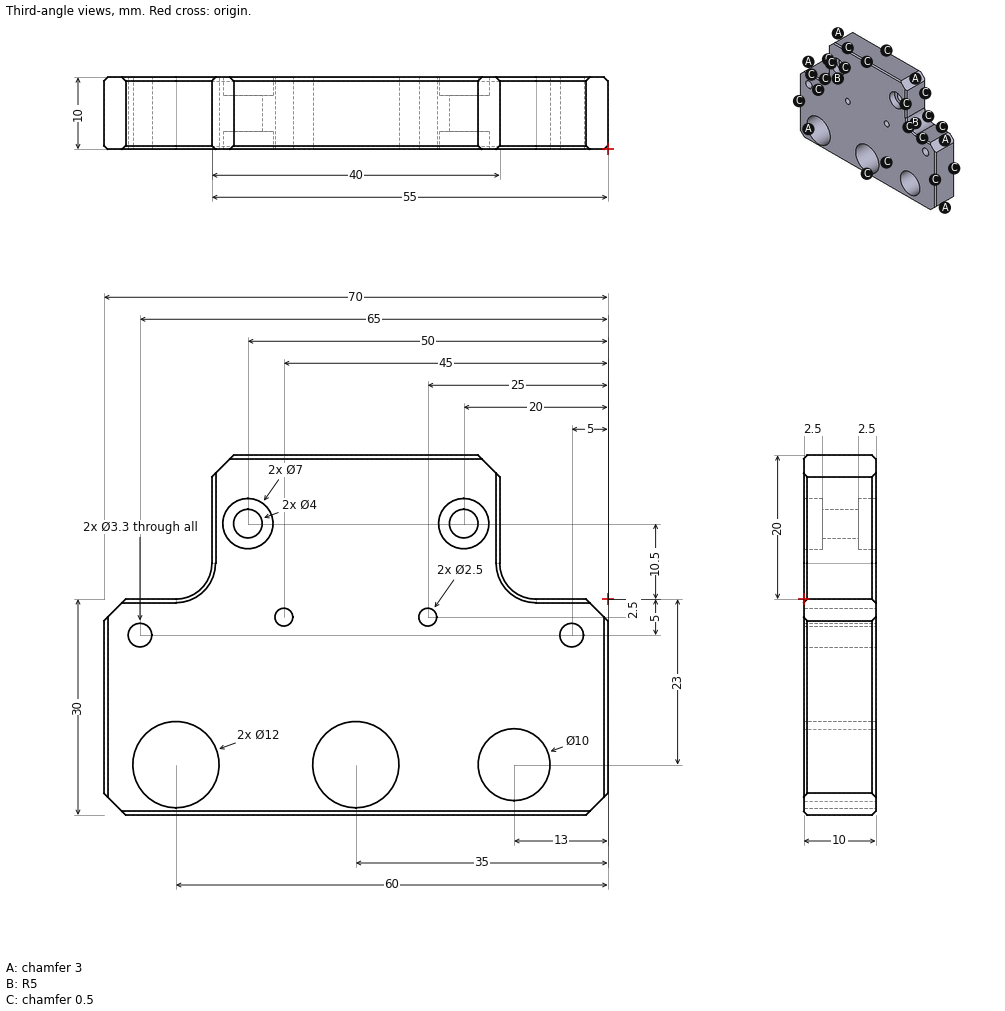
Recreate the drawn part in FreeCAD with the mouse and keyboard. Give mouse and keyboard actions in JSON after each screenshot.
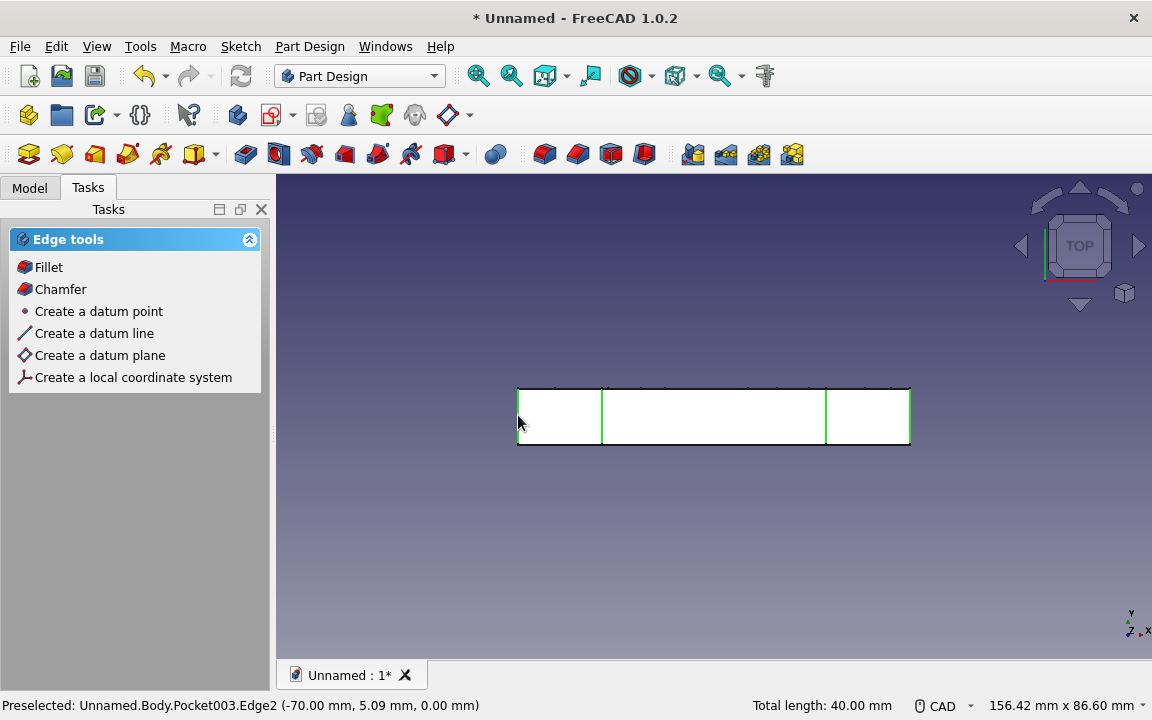
{"action": "key", "text": "1"}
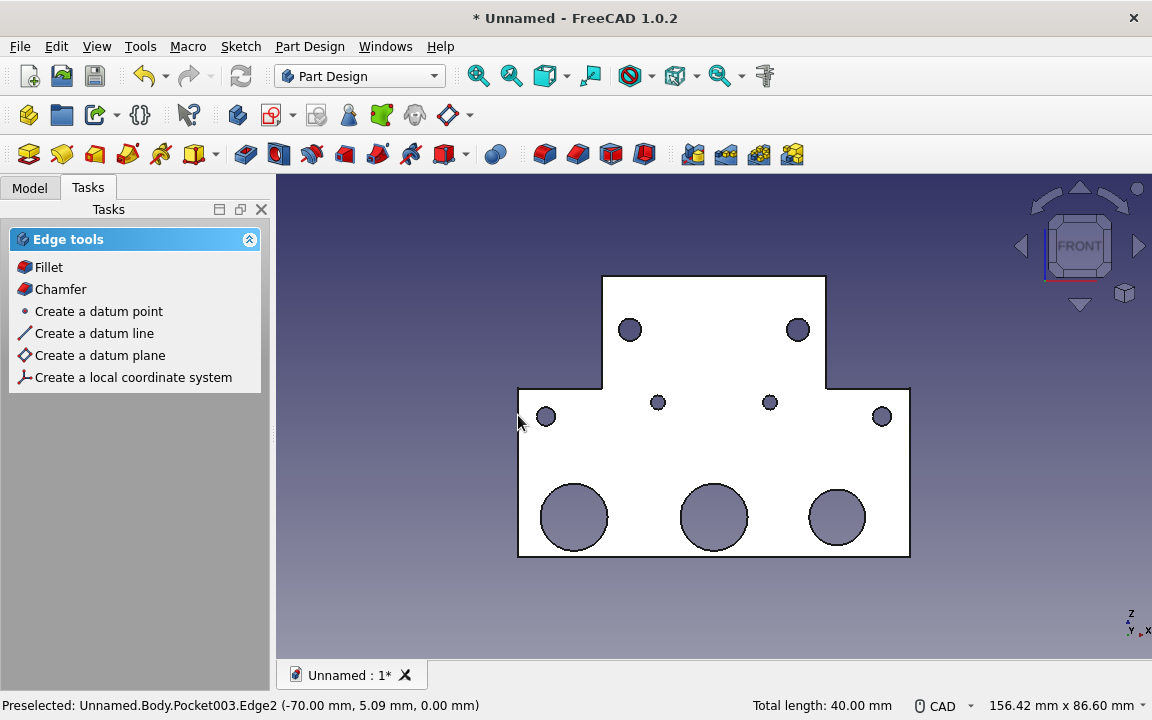
{"action": "key", "text": "3"}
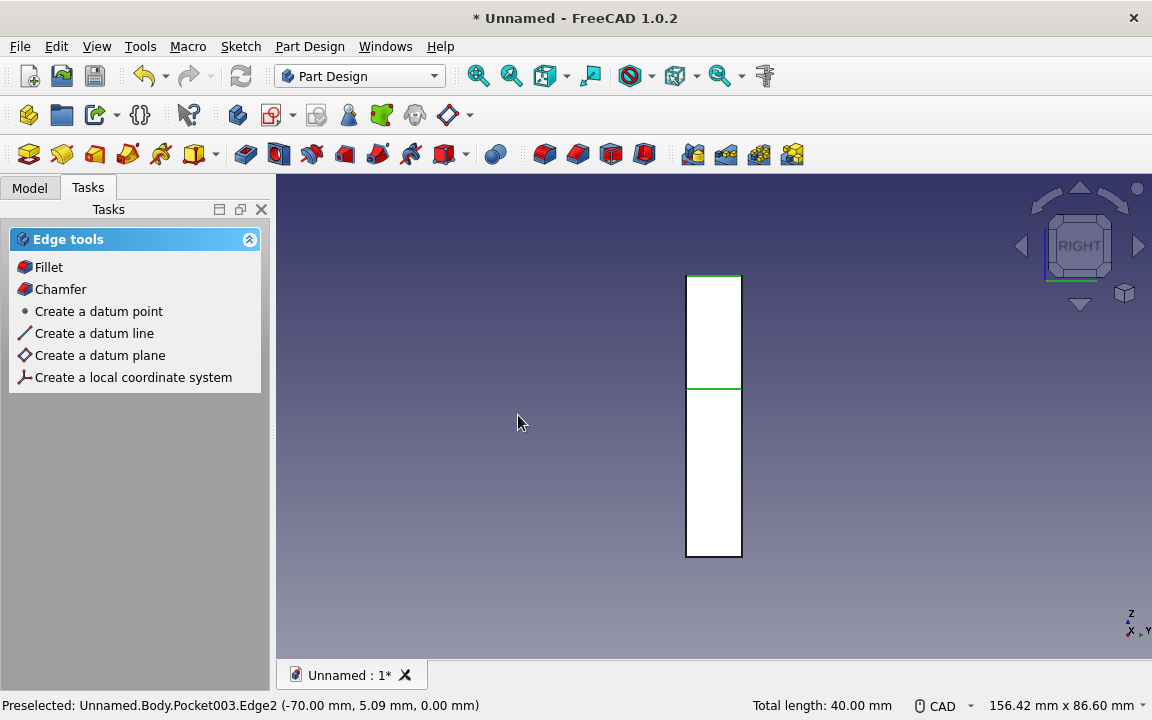
{"action": "key", "text": "5"}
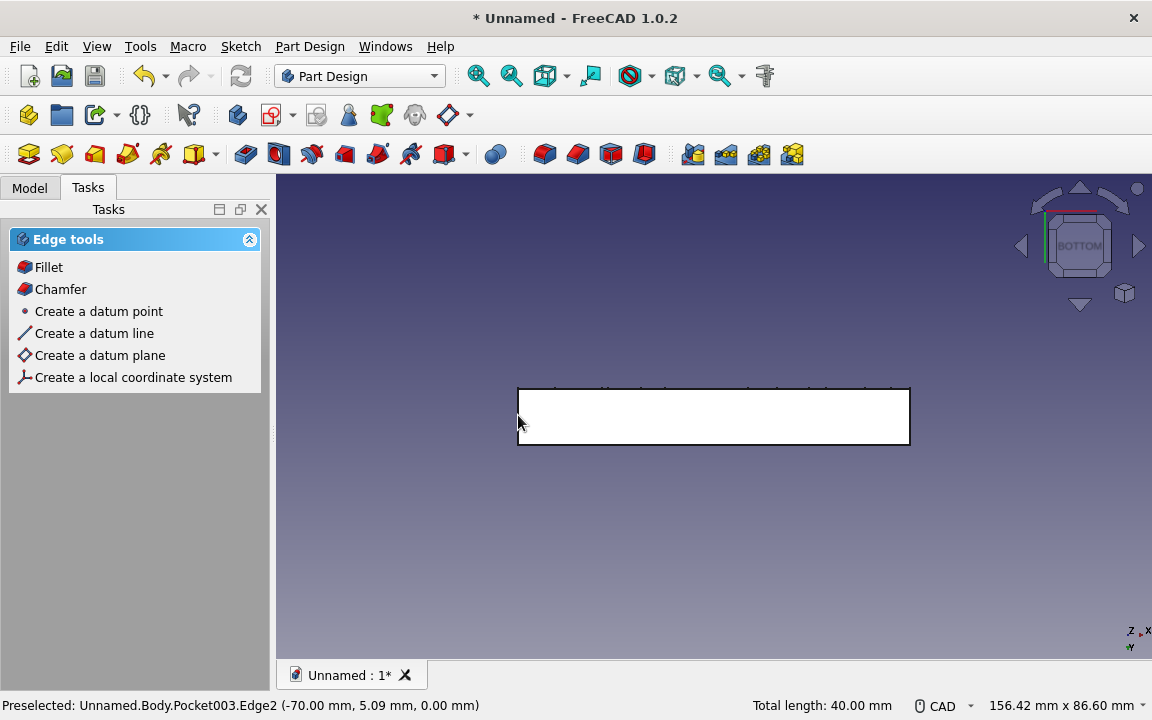
{"action": "left_click", "coordinate": [479, 76]}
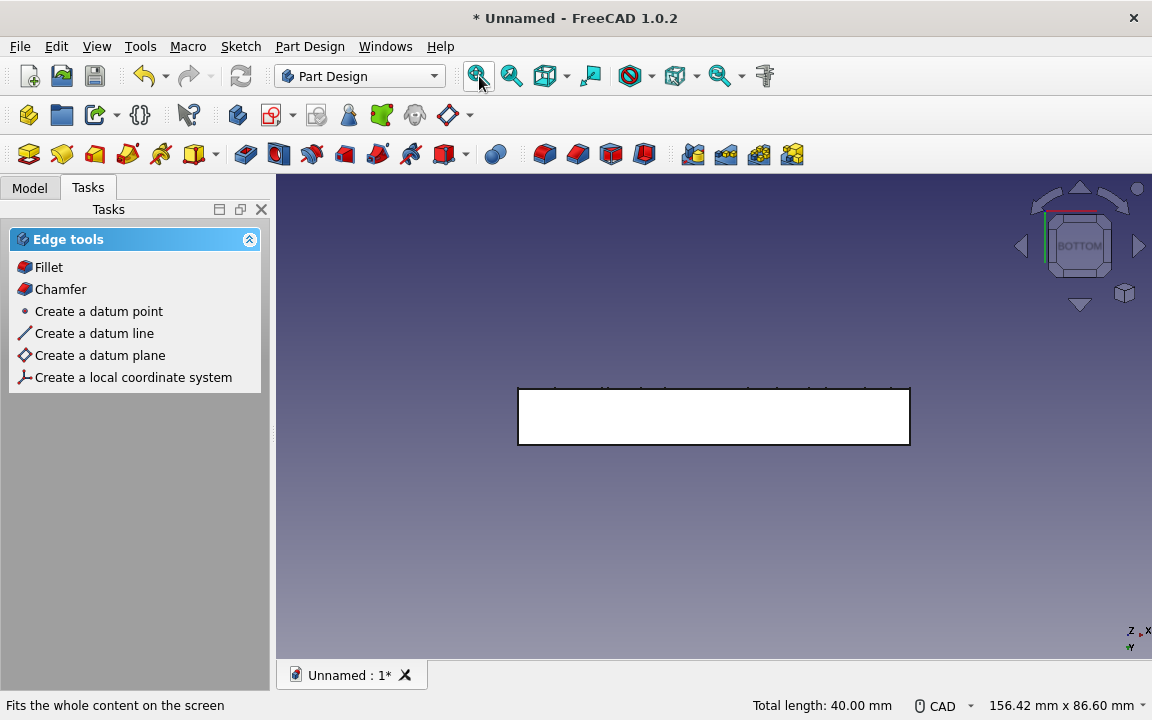
{"action": "left_click", "coordinate": [910, 415], "text": "ctrl"}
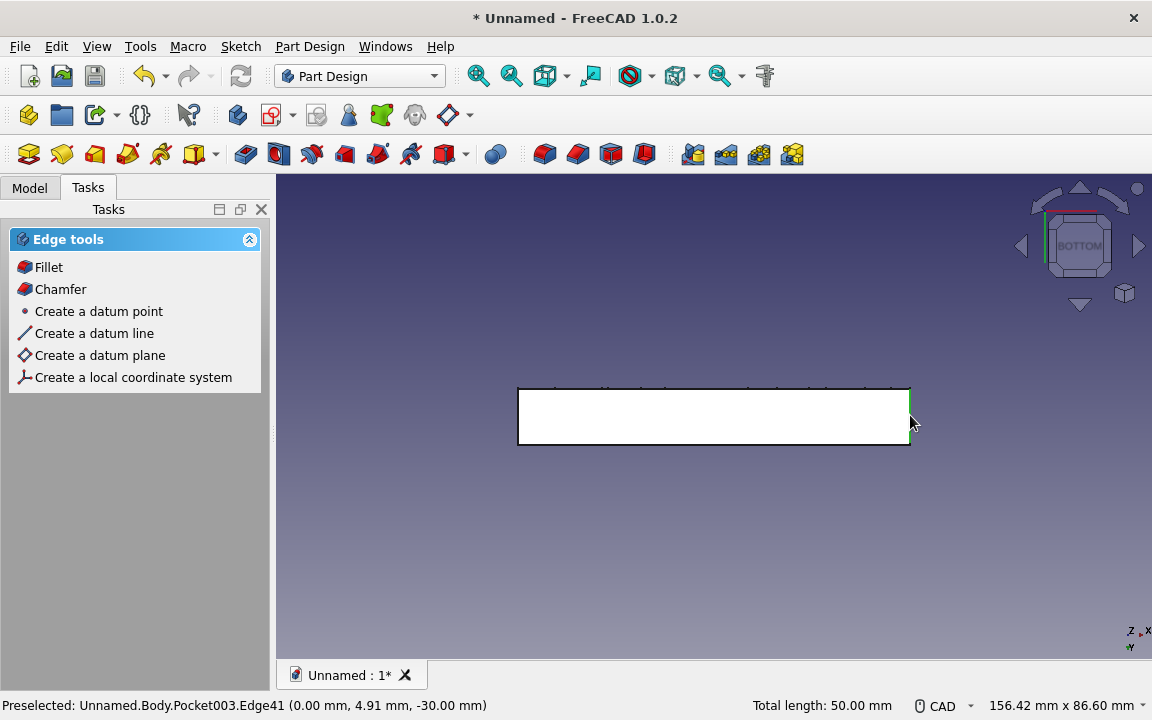
{"action": "left_click", "coordinate": [518, 415], "text": "ctrl"}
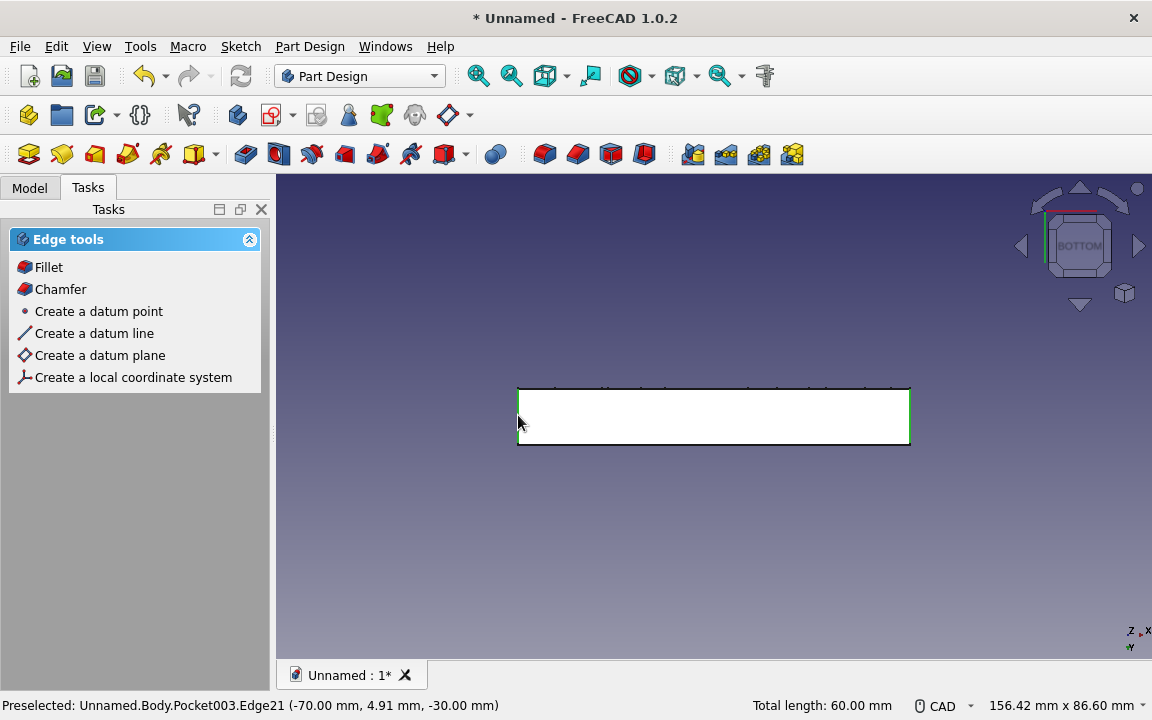
{"action": "left_click", "coordinate": [578, 154]}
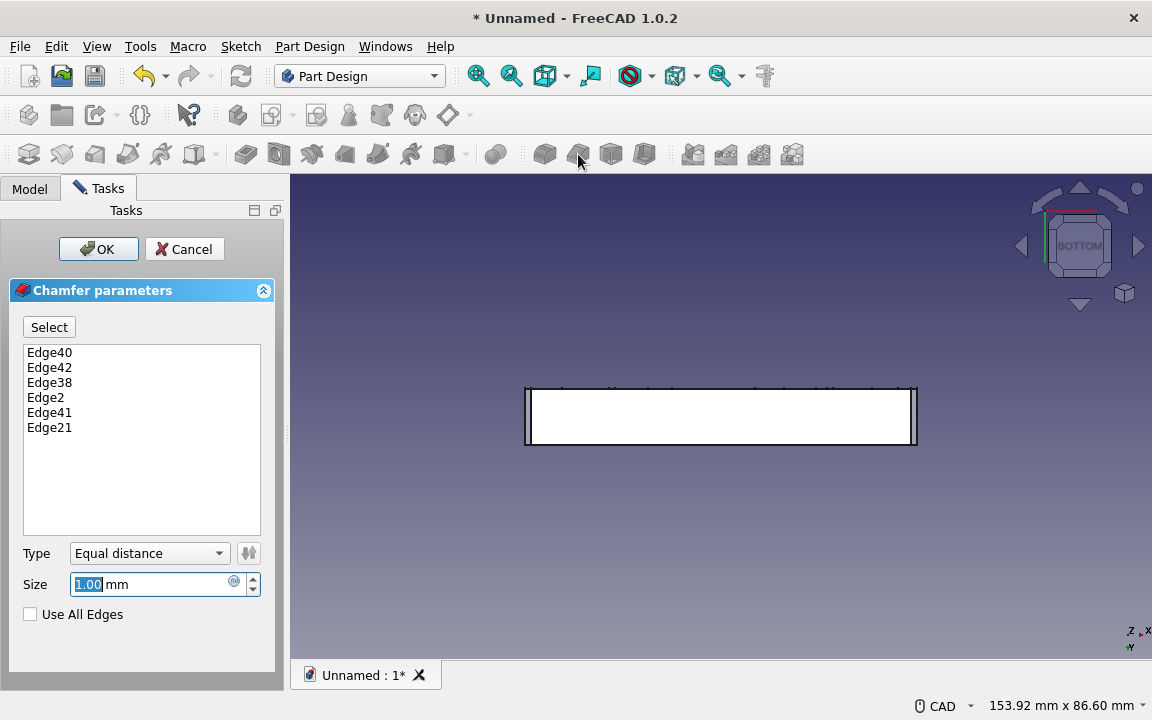
{"action": "type", "text": "3"}
{"action": "key", "text": "Tab"}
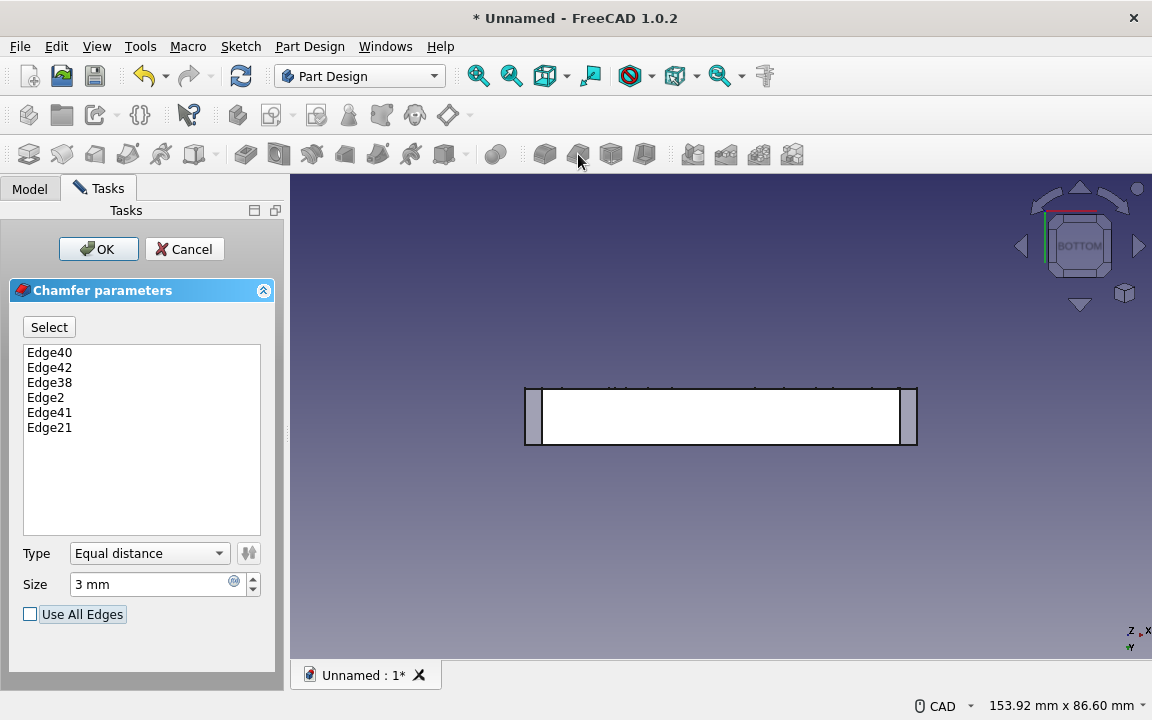
{"action": "left_click", "coordinate": [99, 249]}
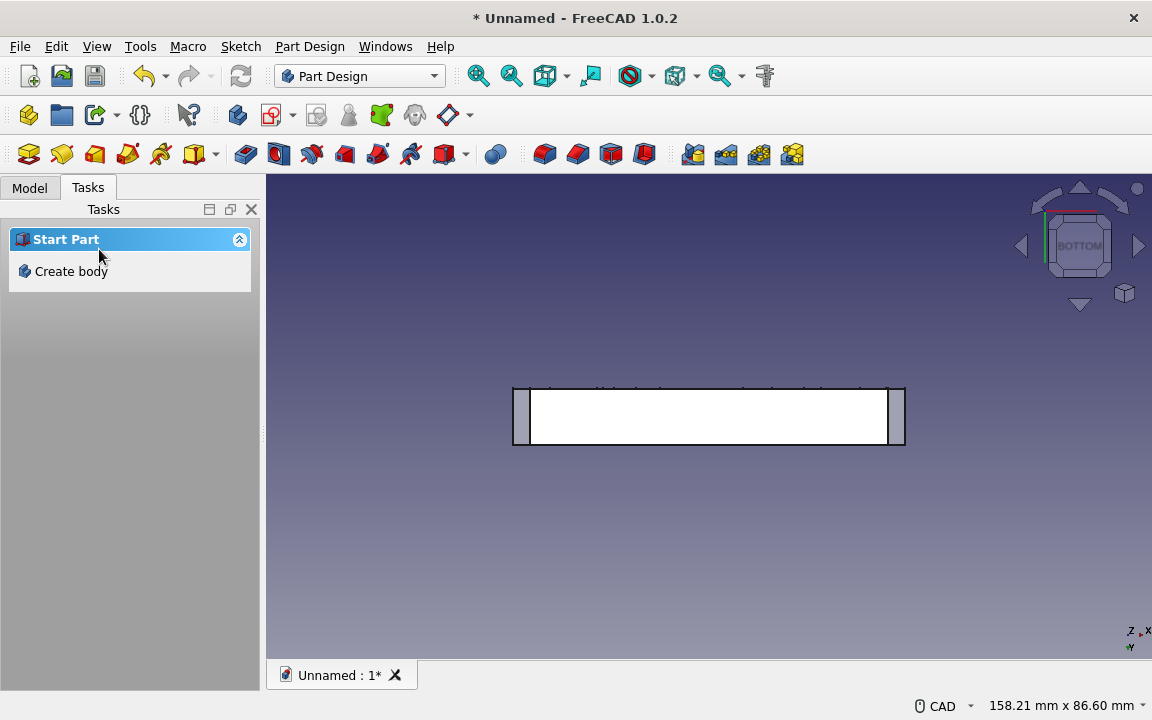
{"action": "left_click", "coordinate": [479, 76]}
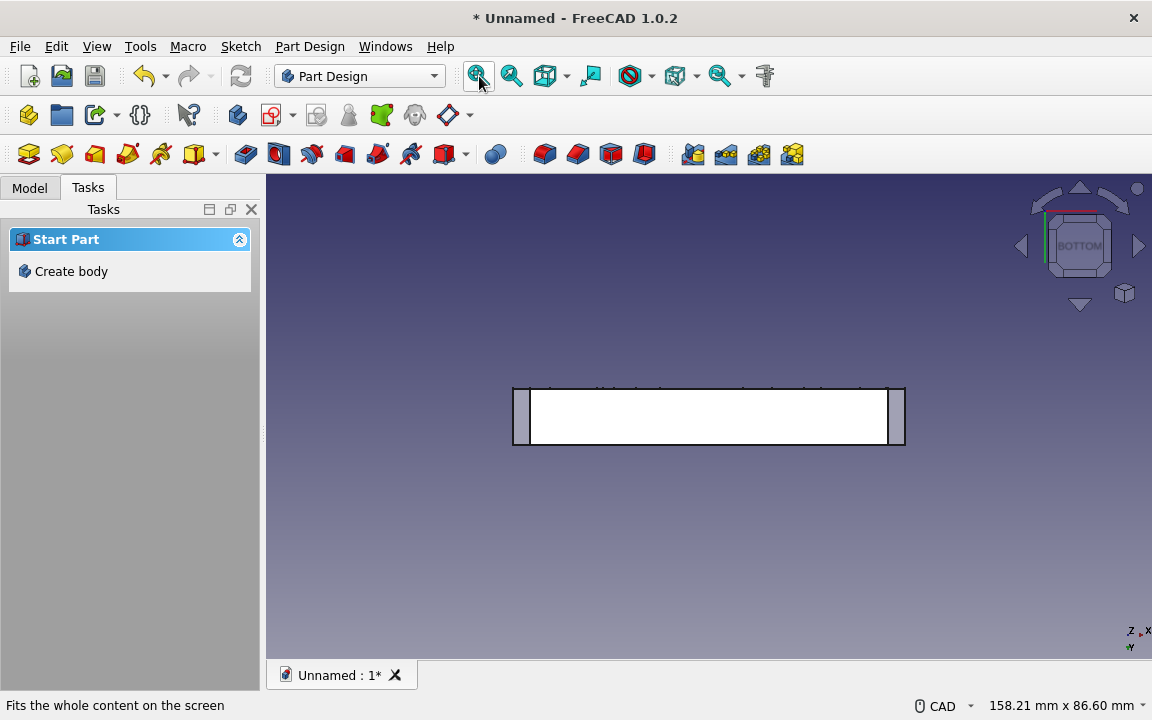
{"action": "key", "text": "0"}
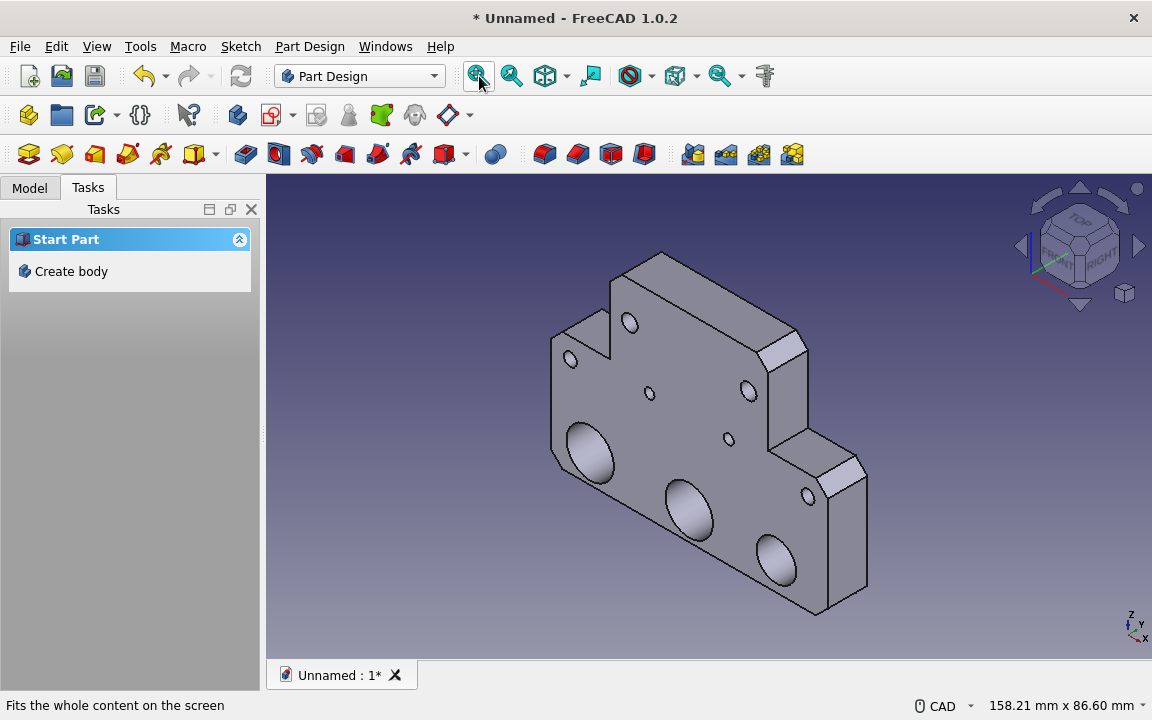
{"action": "key", "text": "2"}